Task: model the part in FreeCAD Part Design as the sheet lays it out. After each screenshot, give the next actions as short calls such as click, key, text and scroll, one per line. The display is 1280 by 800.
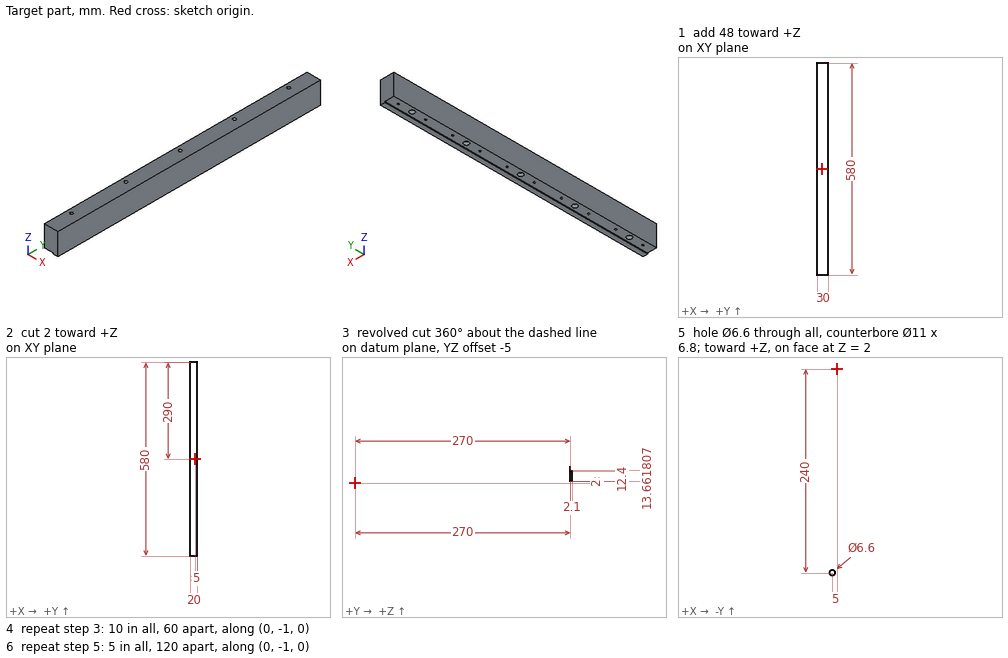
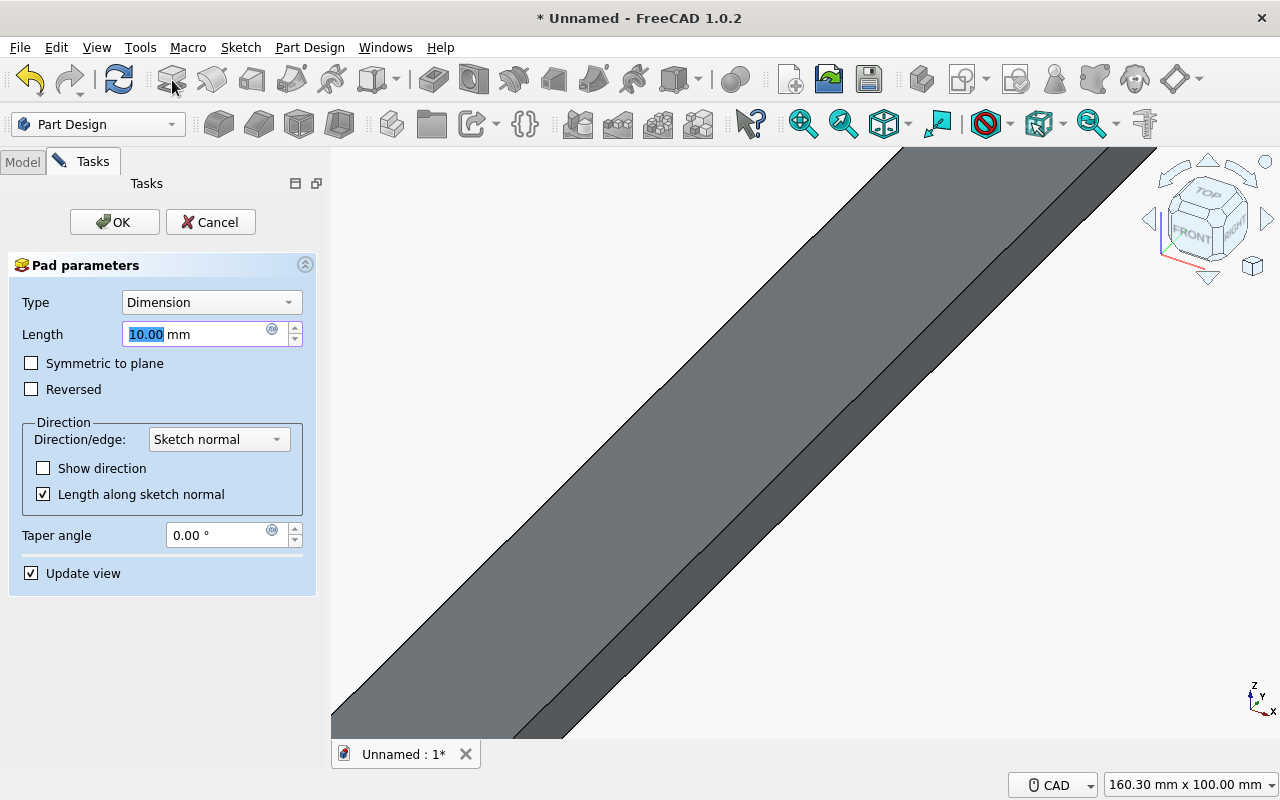
text(48)
key(Tab)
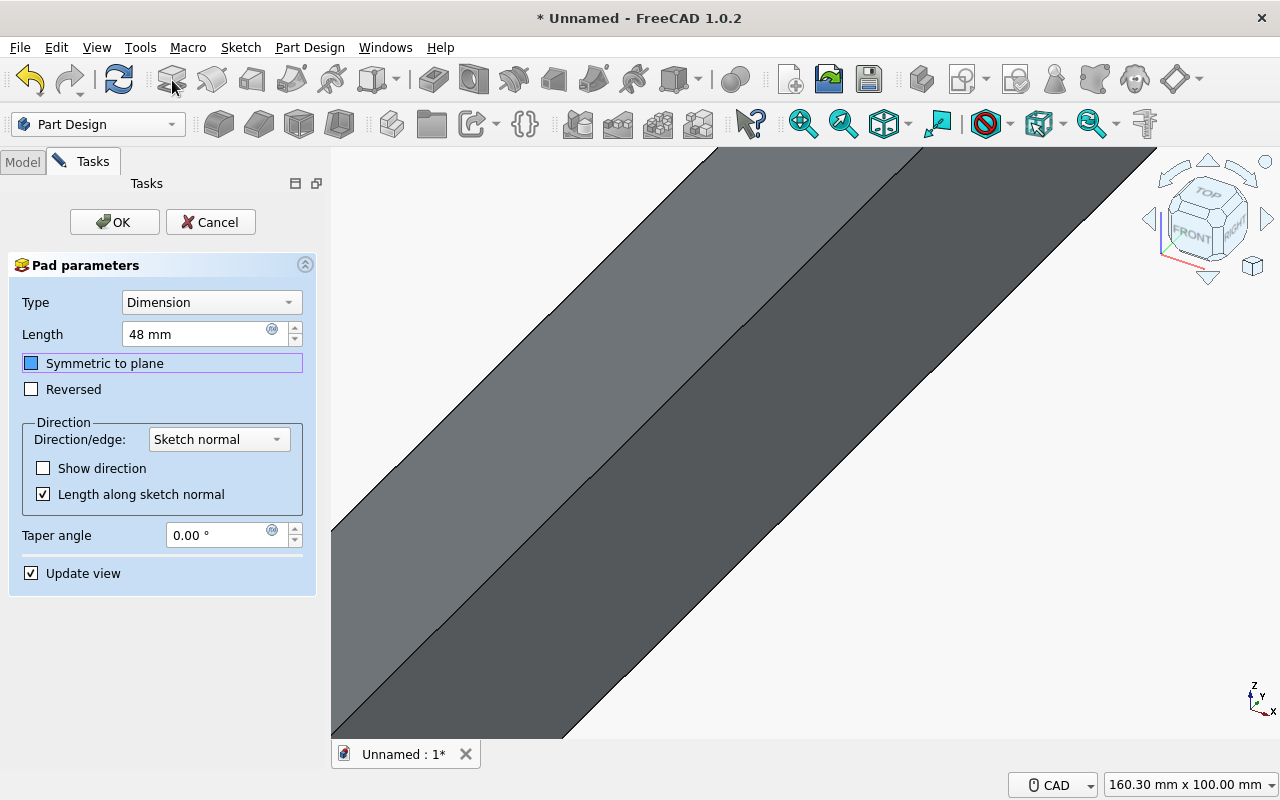
click(115, 222)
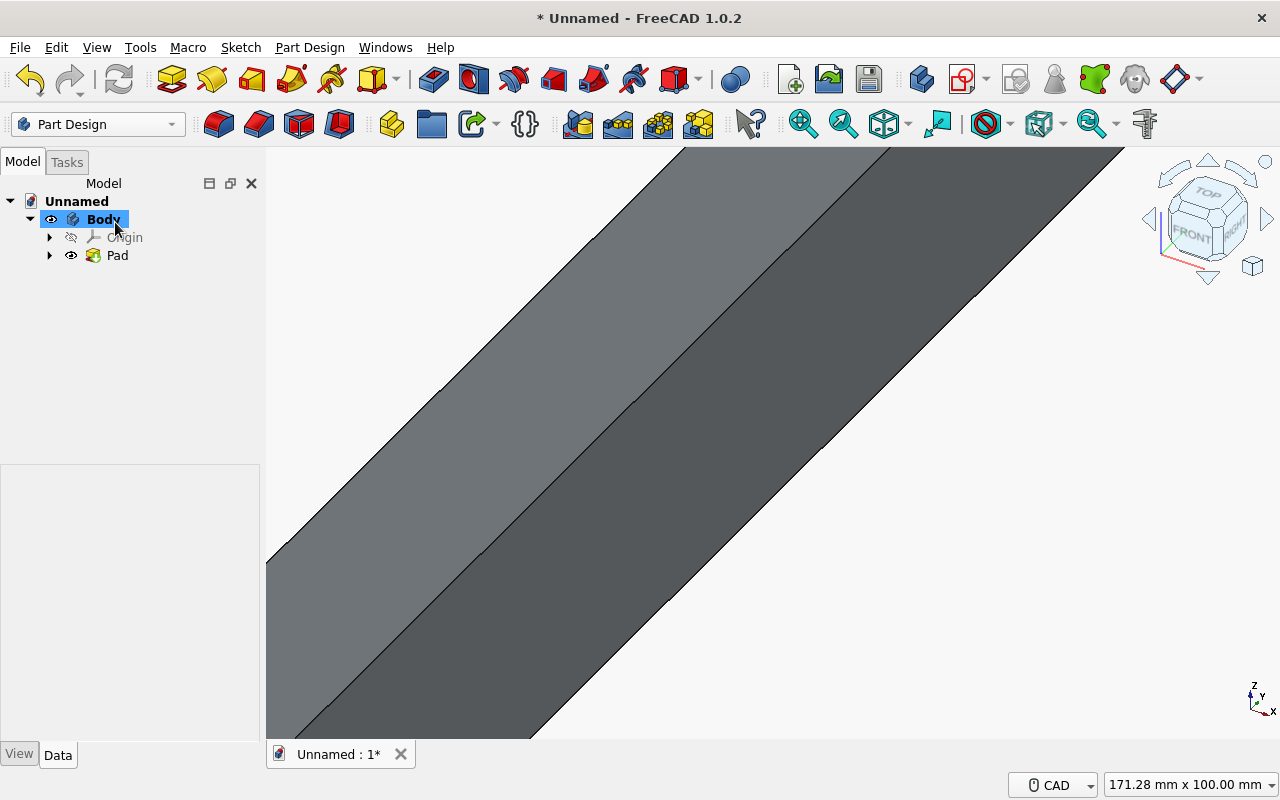
key(v)
key(f)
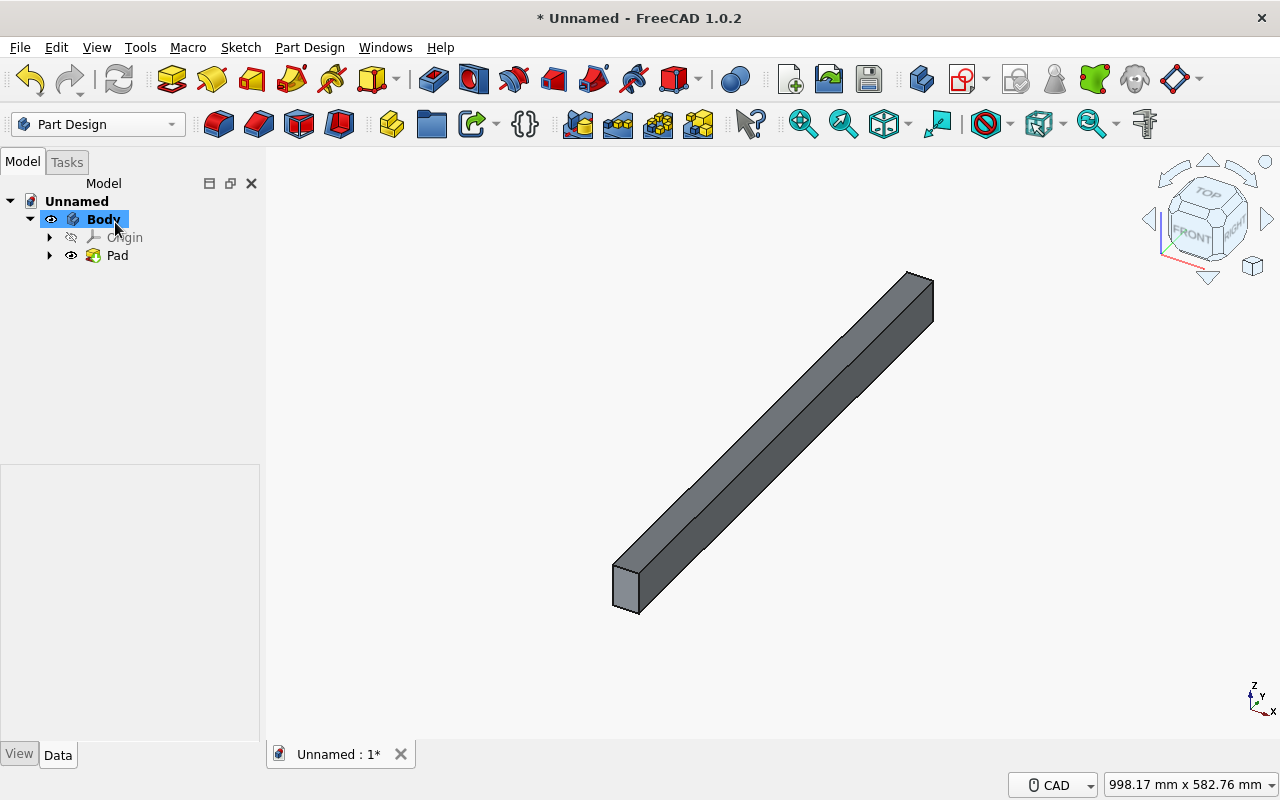
click(962, 80)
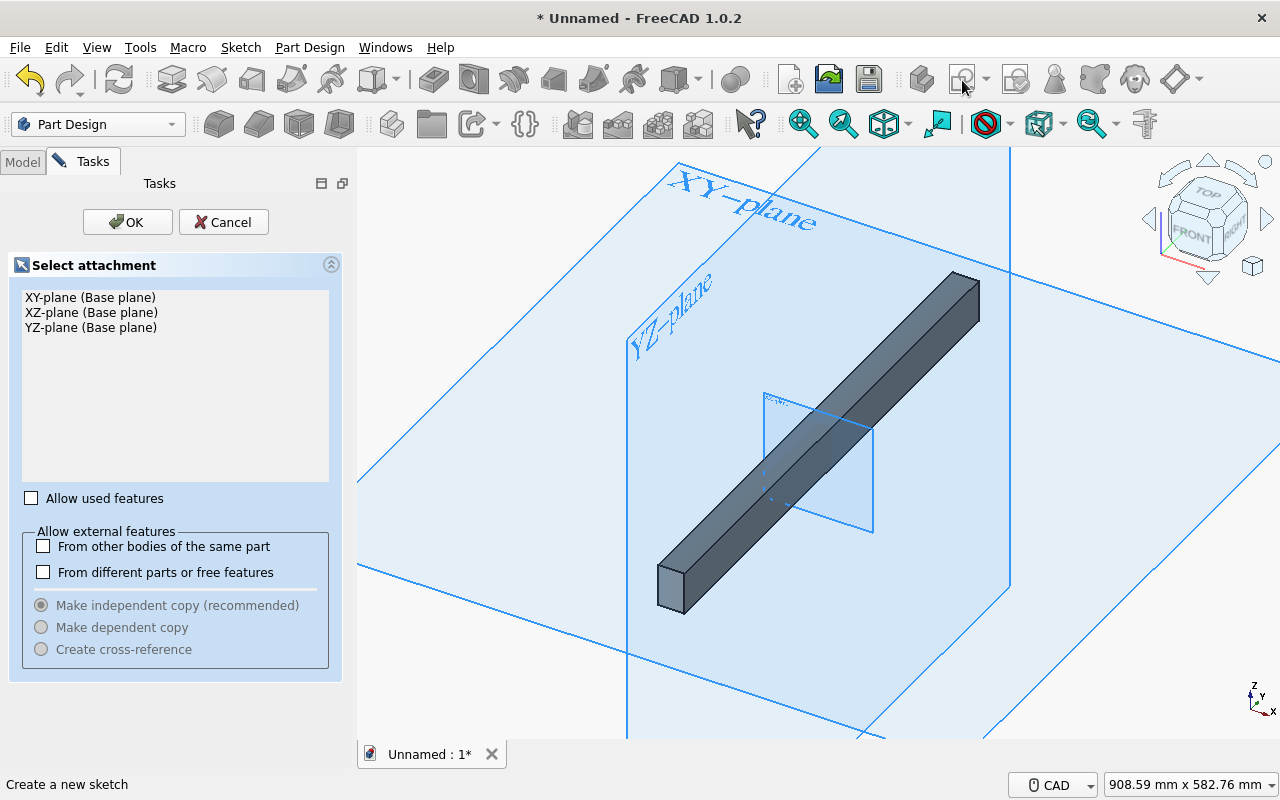
click(82, 298)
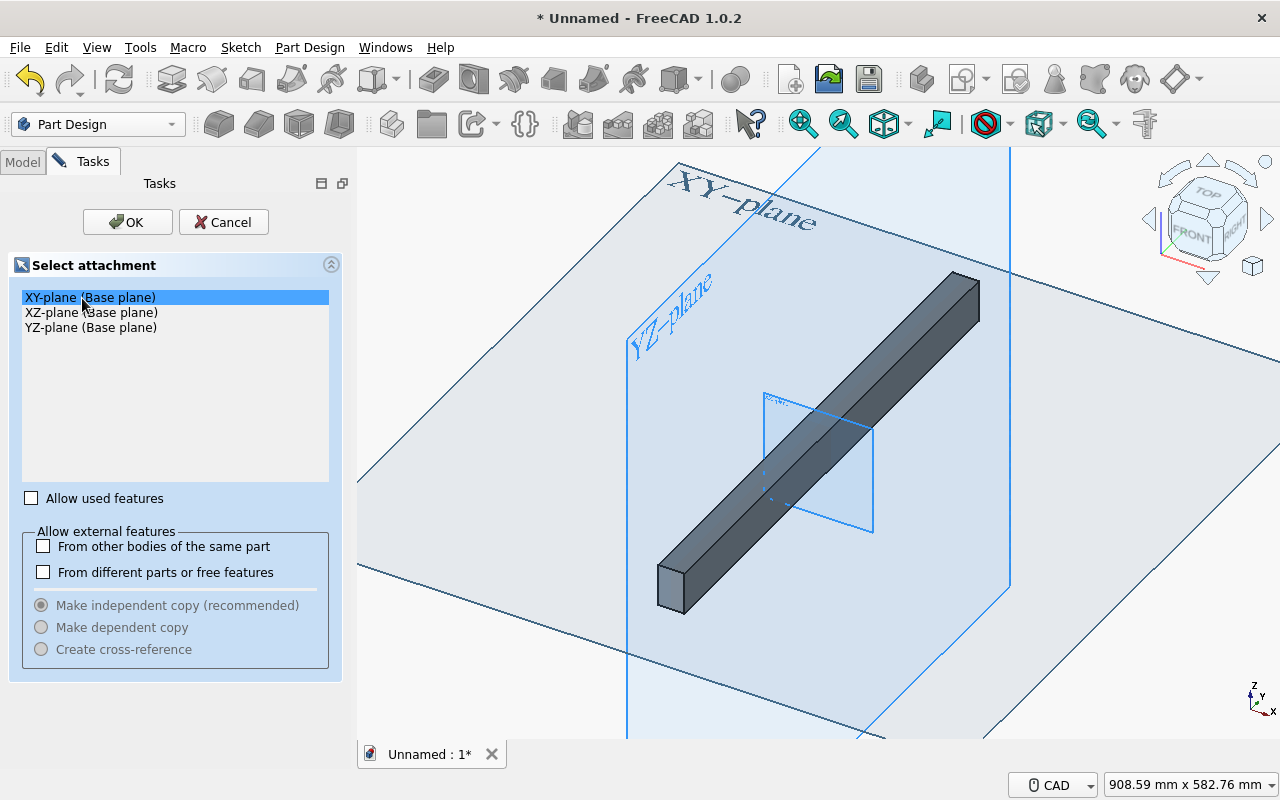
click(128, 222)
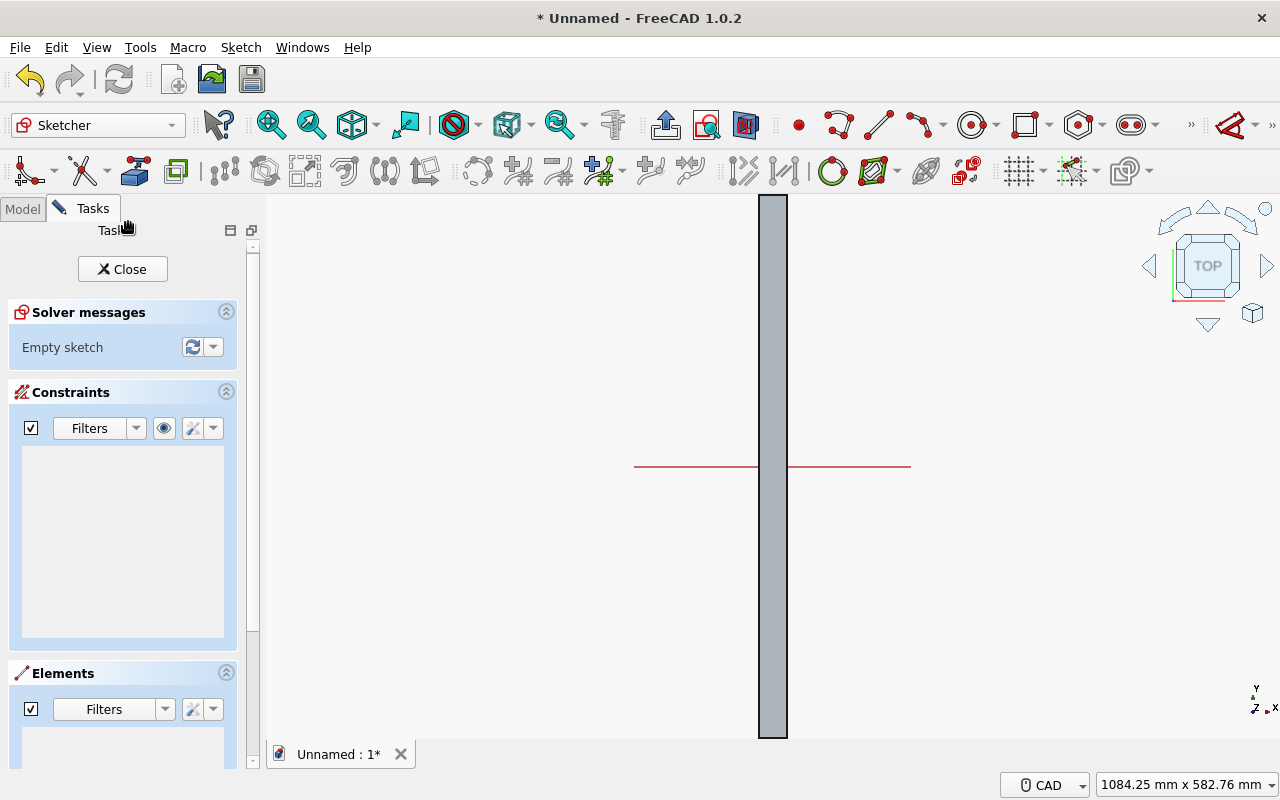
key(q)
key(s)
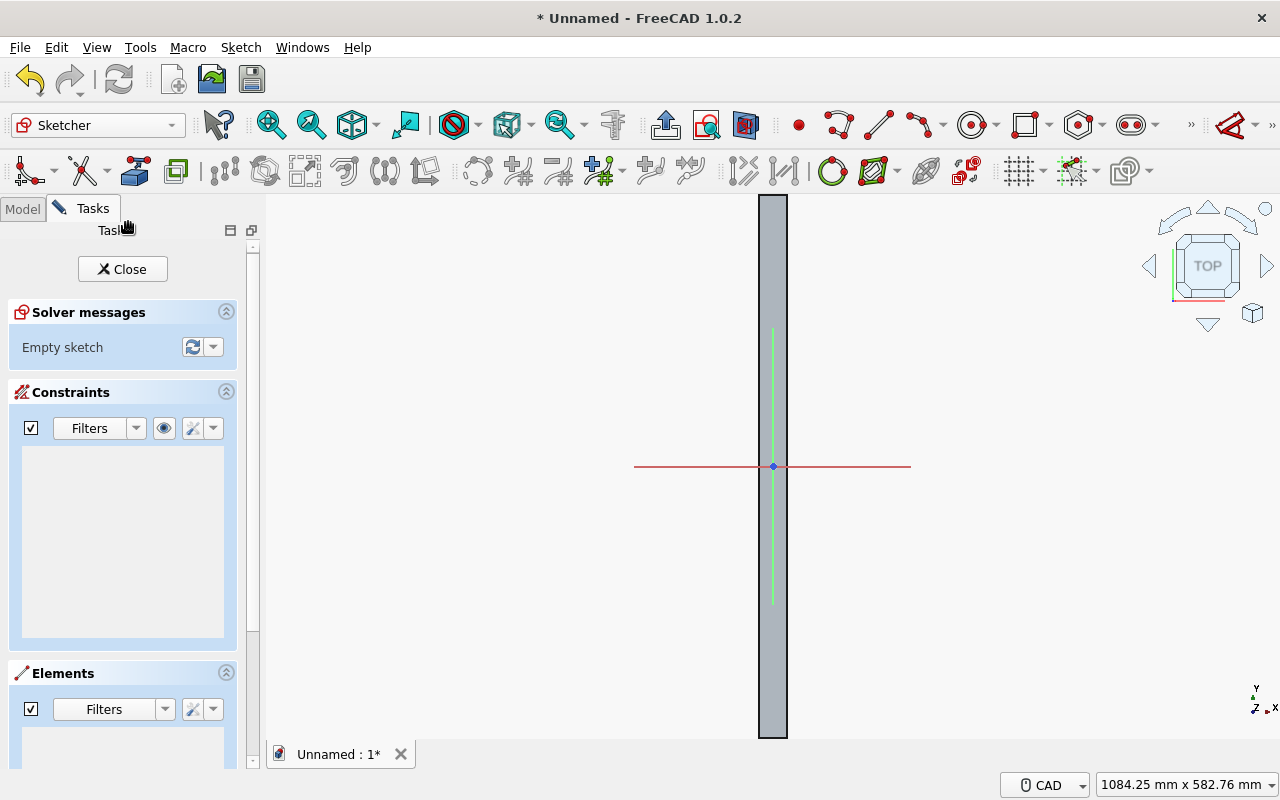
scroll(575, 466, down, 2)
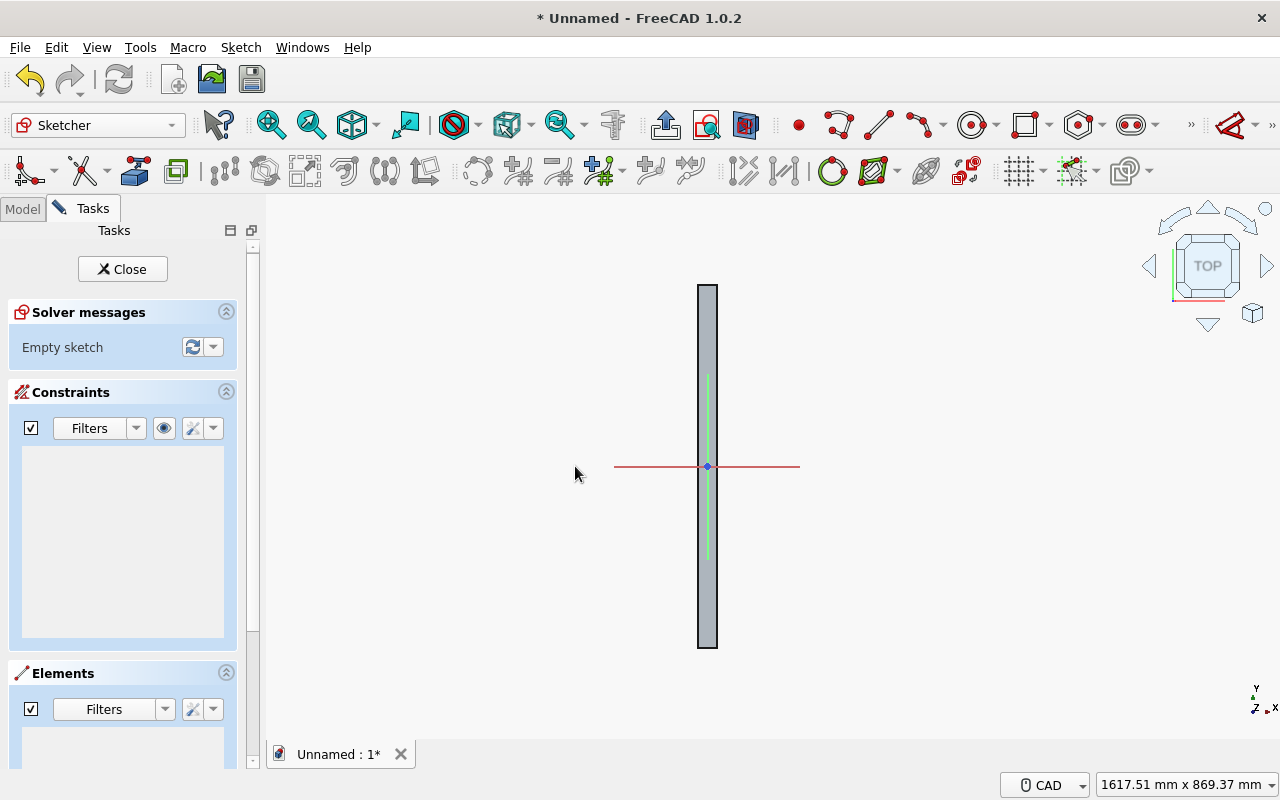
key(g)
key(r)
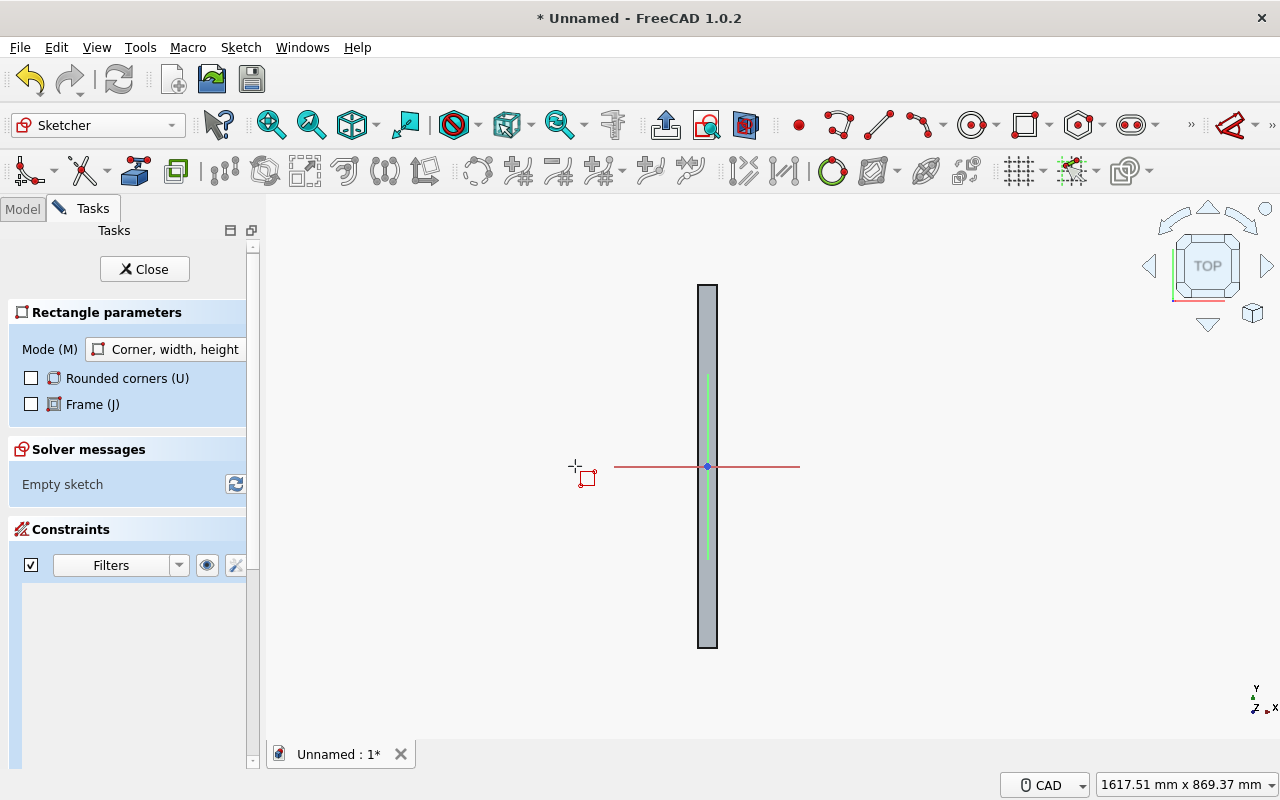
scroll(698, 285, up, 3)